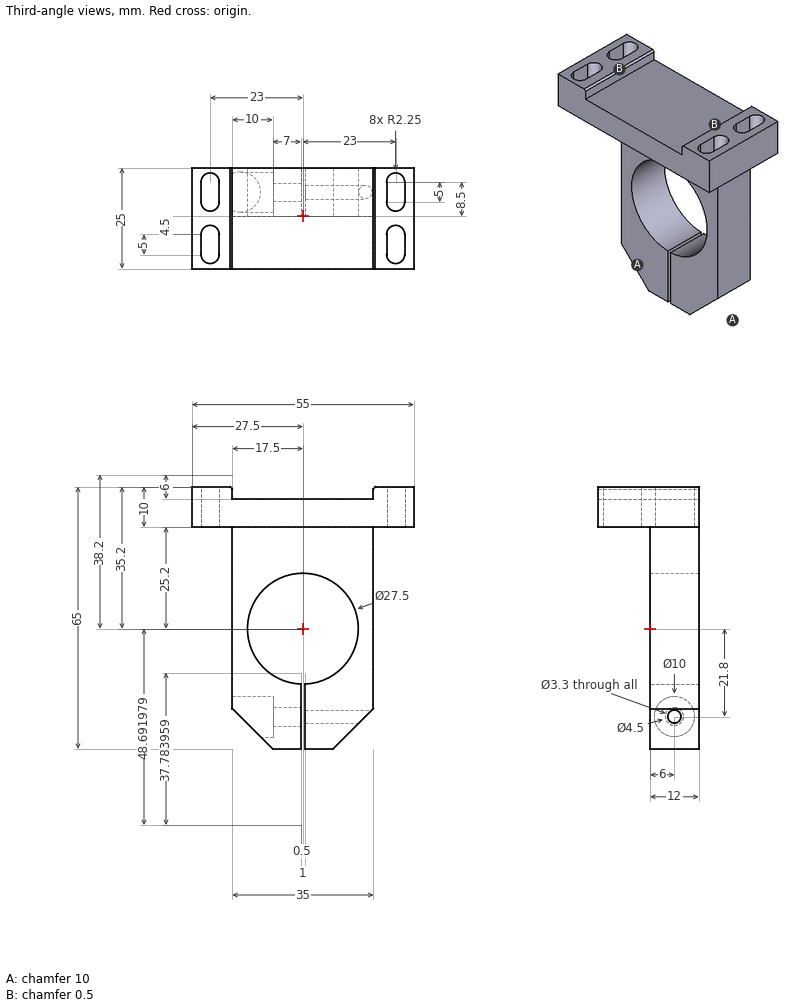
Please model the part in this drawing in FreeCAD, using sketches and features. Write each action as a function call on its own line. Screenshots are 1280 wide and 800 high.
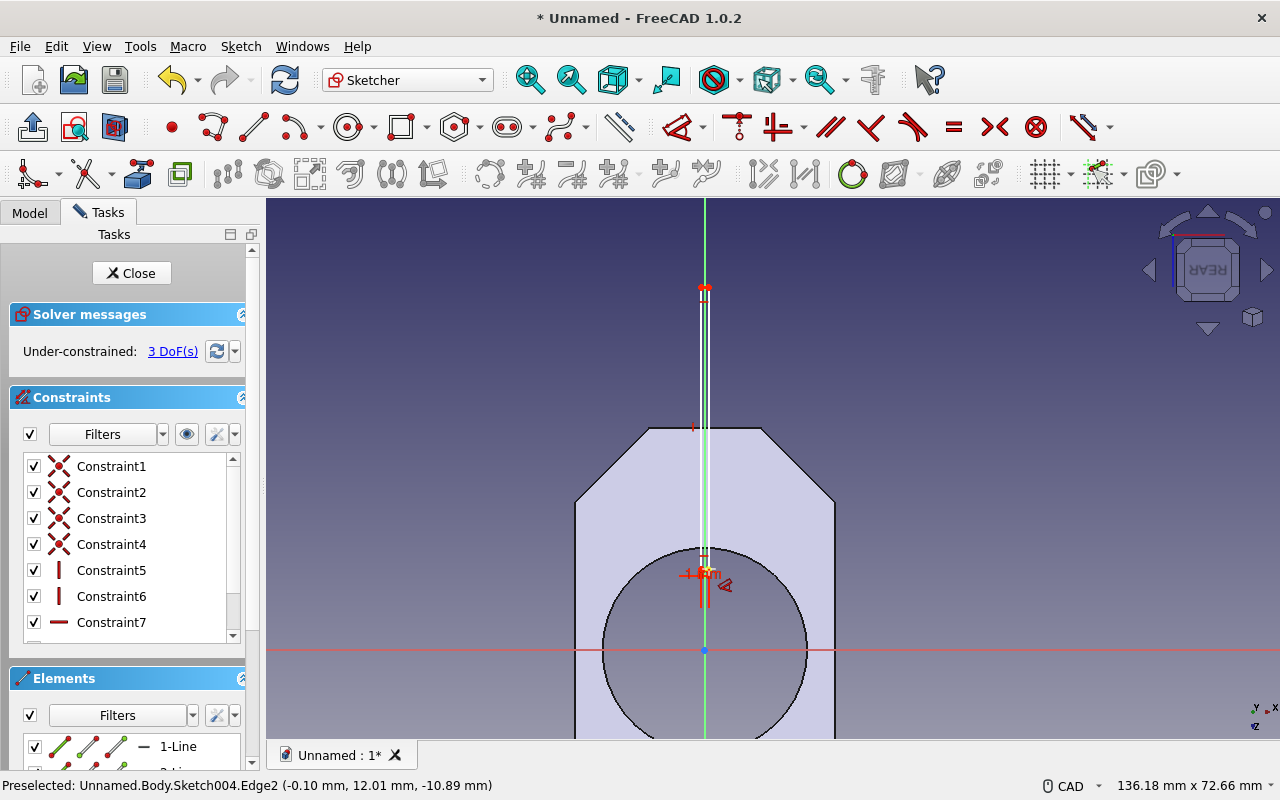
scroll(701, 288, up, 12)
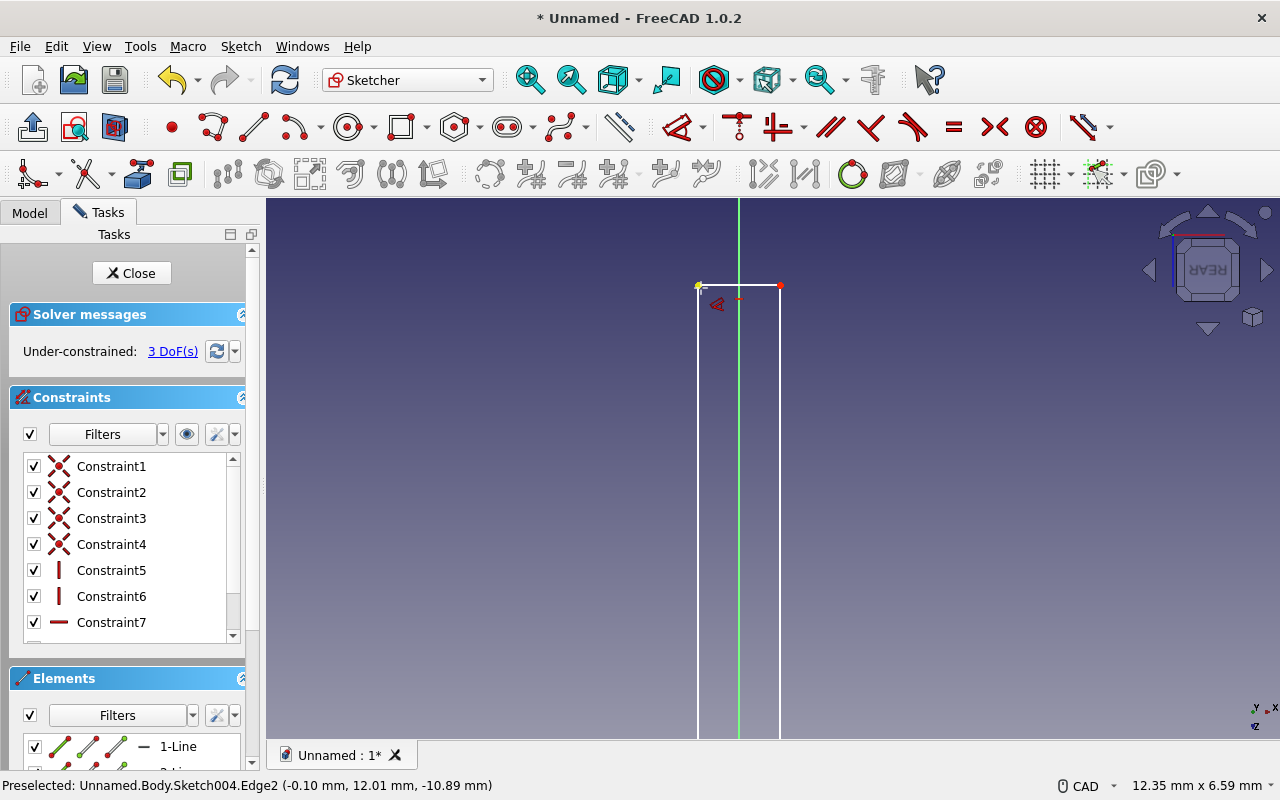
click(698, 285)
click(719, 251)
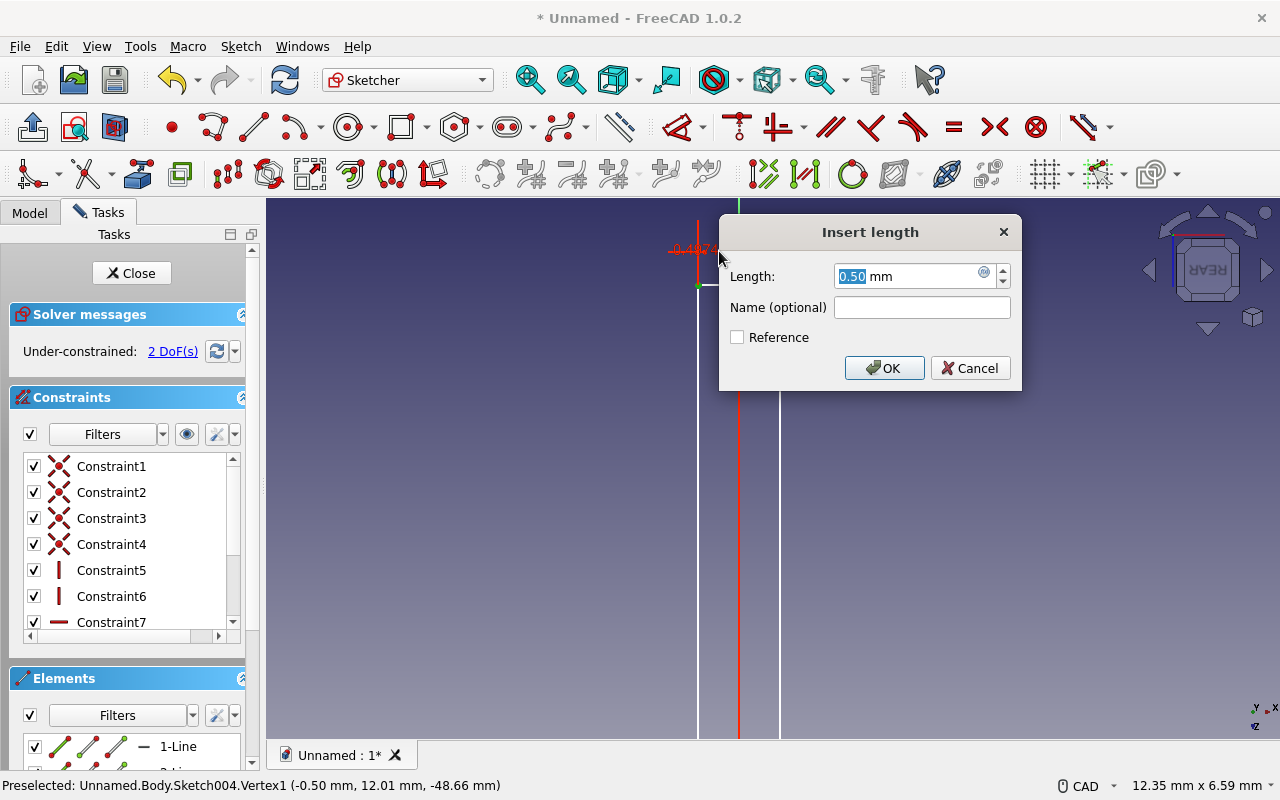
text(0.5)
key(Return)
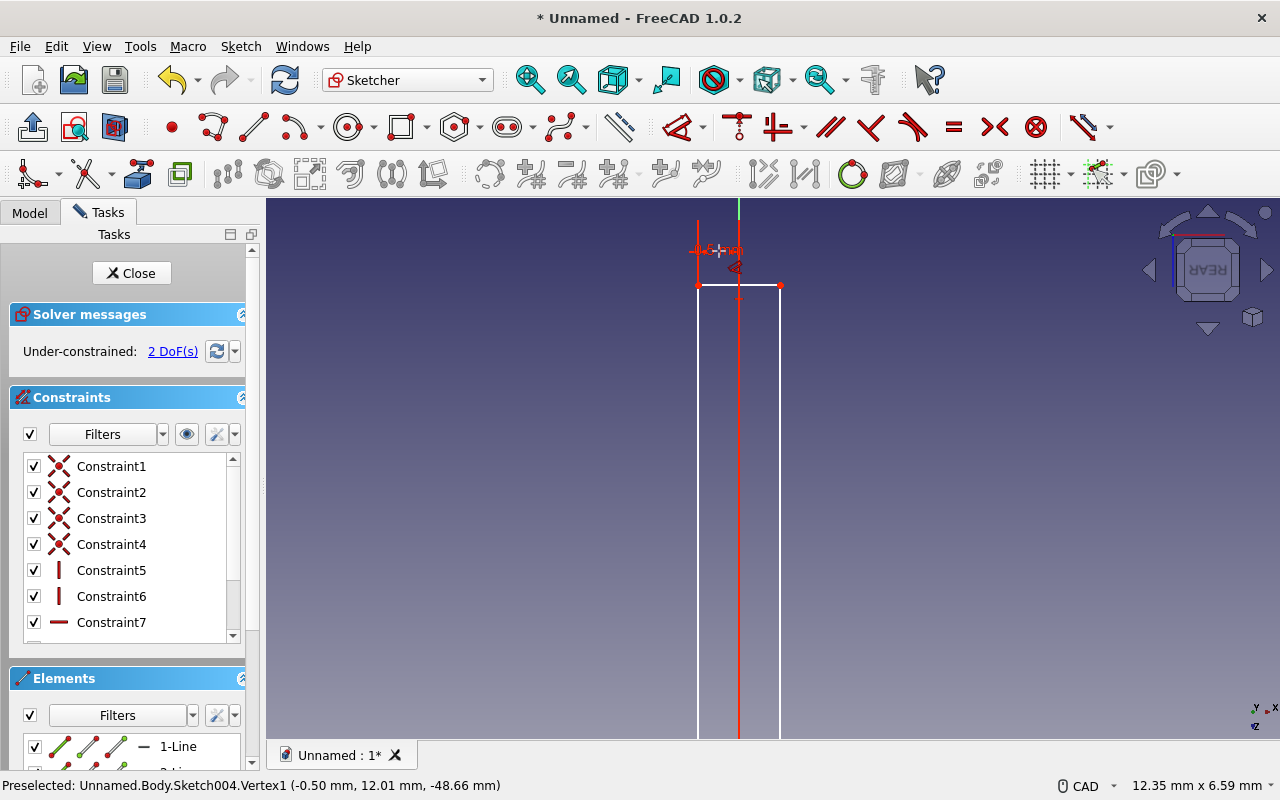
scroll(701, 288, down, 12)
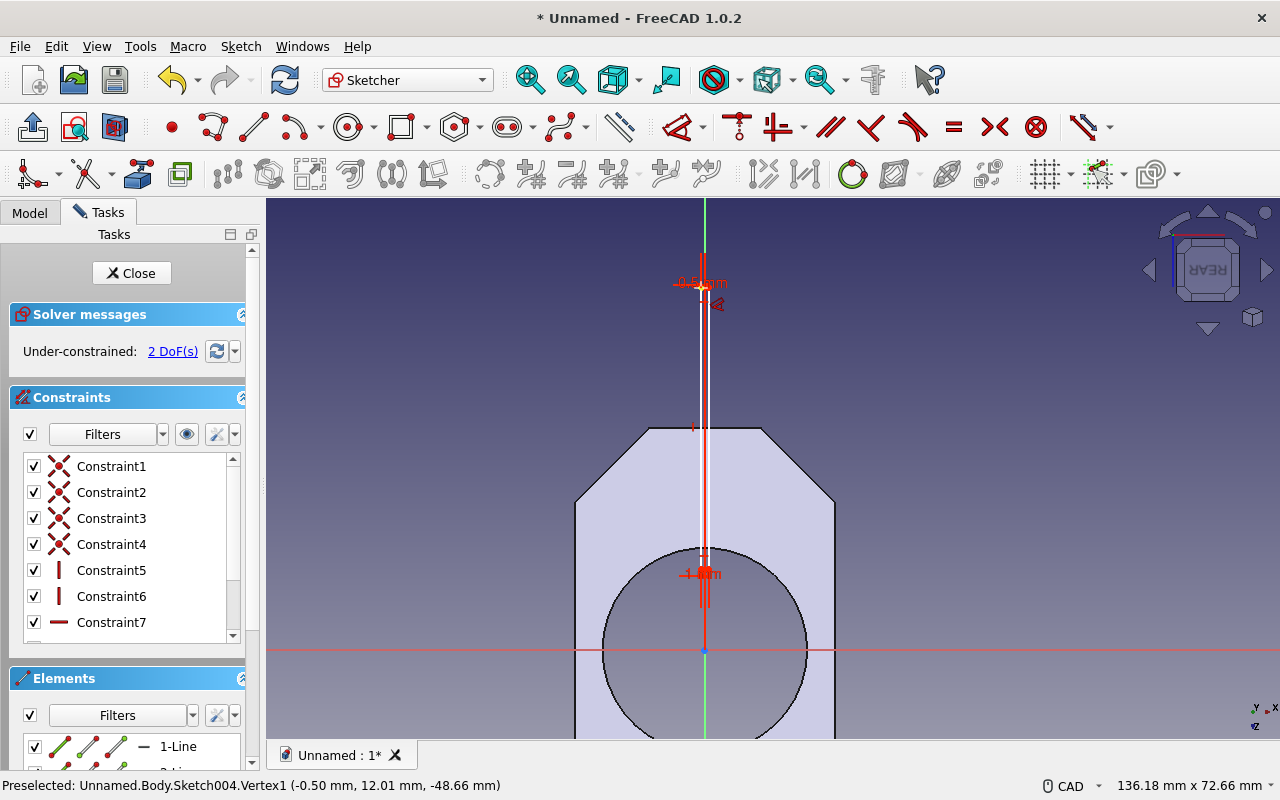
scroll(701, 372, up, 7)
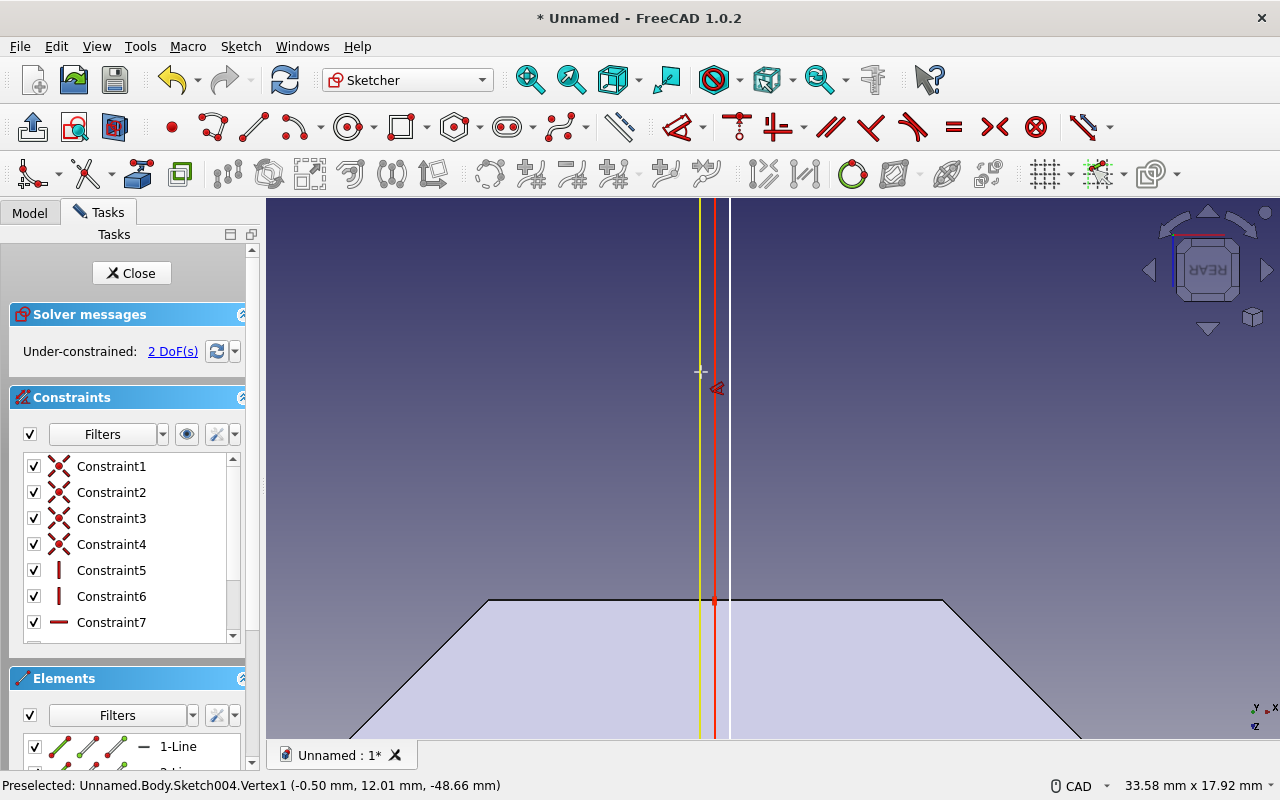
click(700, 372)
click(666, 468)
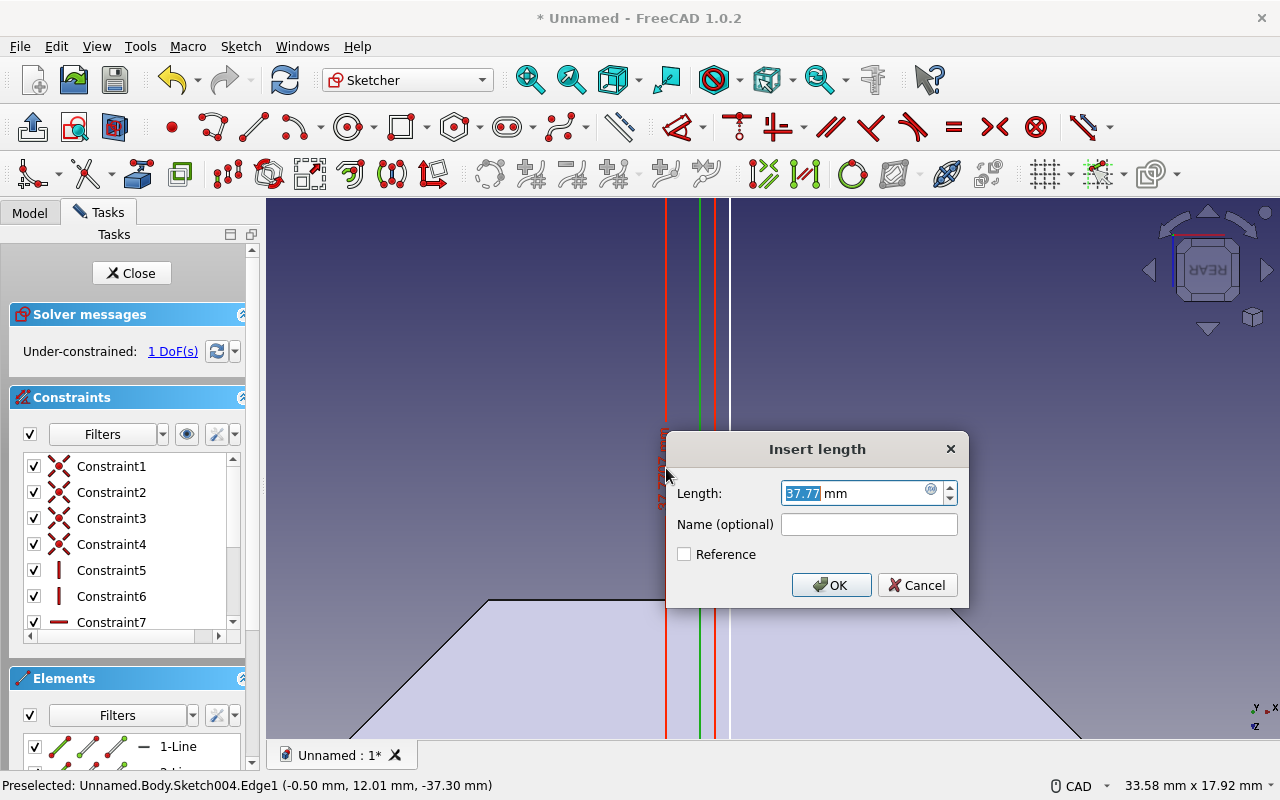
text(37.783959)
key(Return)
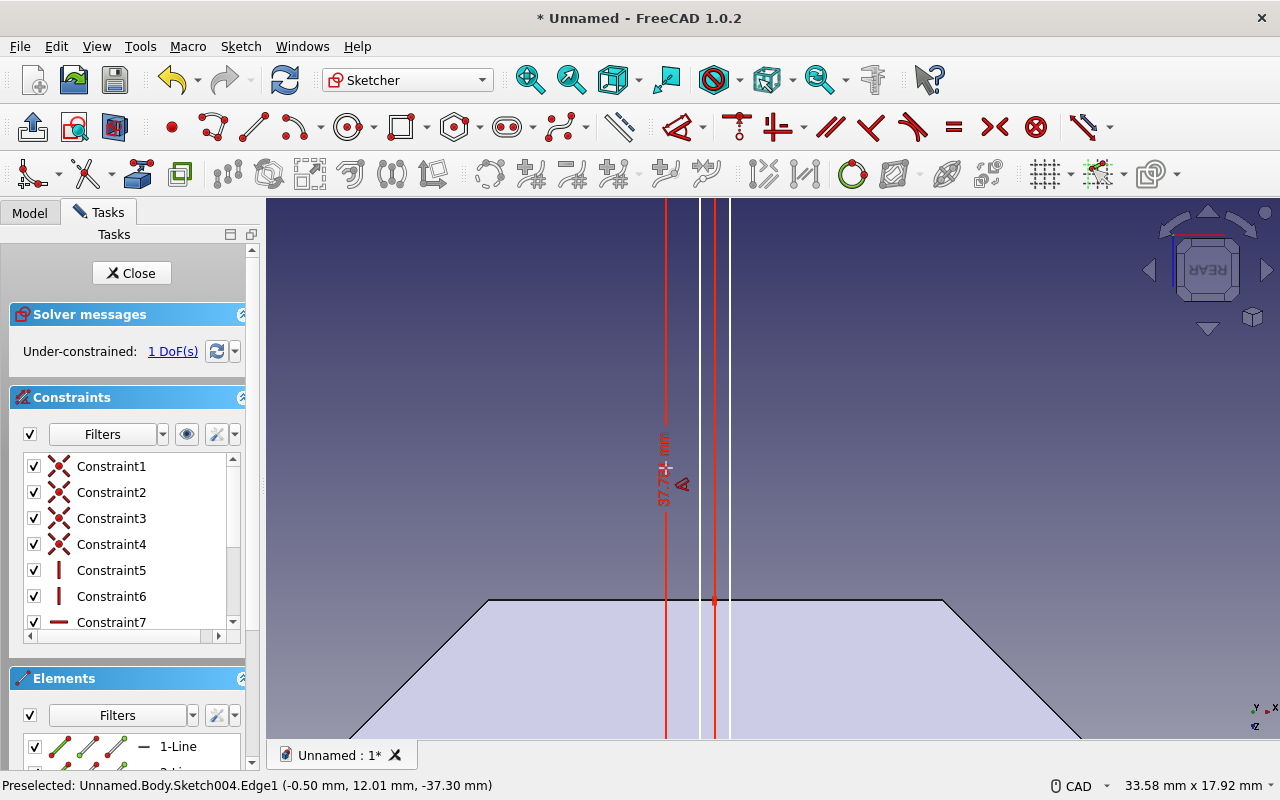
scroll(701, 372, down, 7)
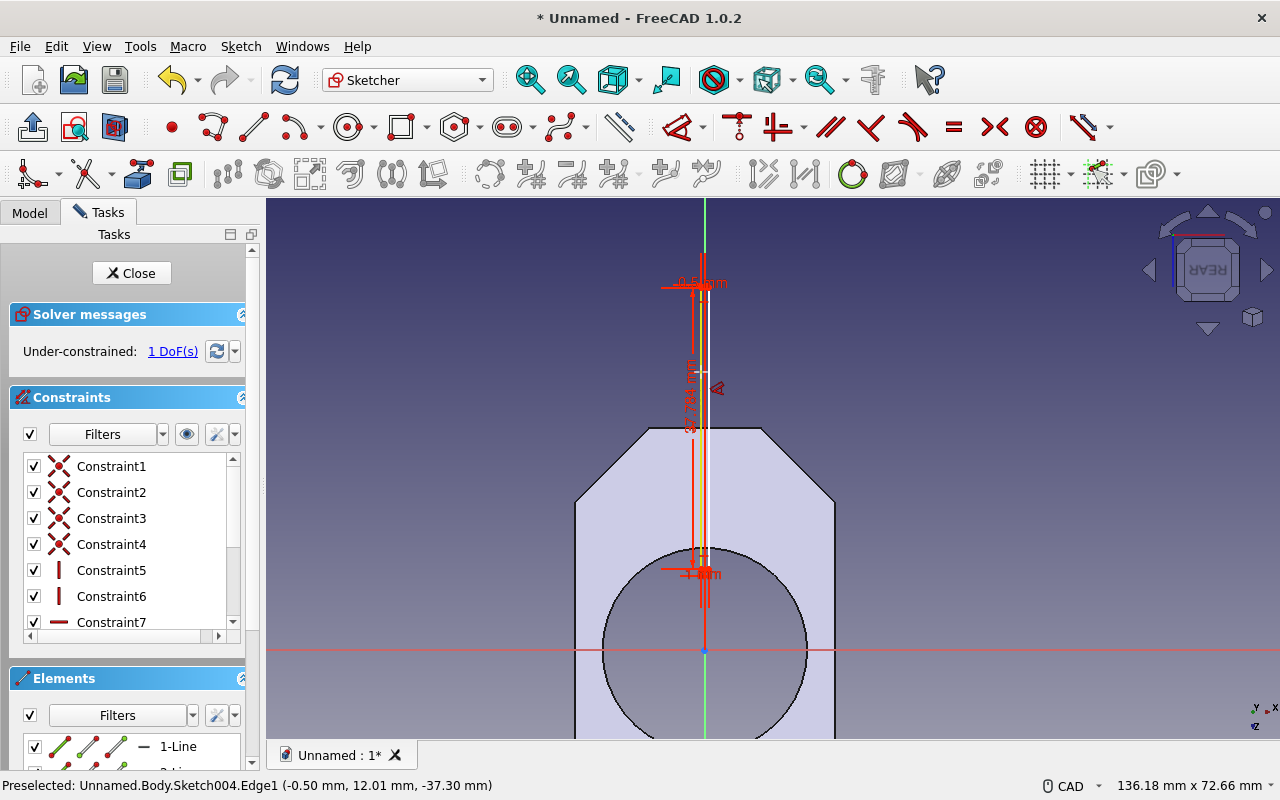
scroll(701, 288, up, 3)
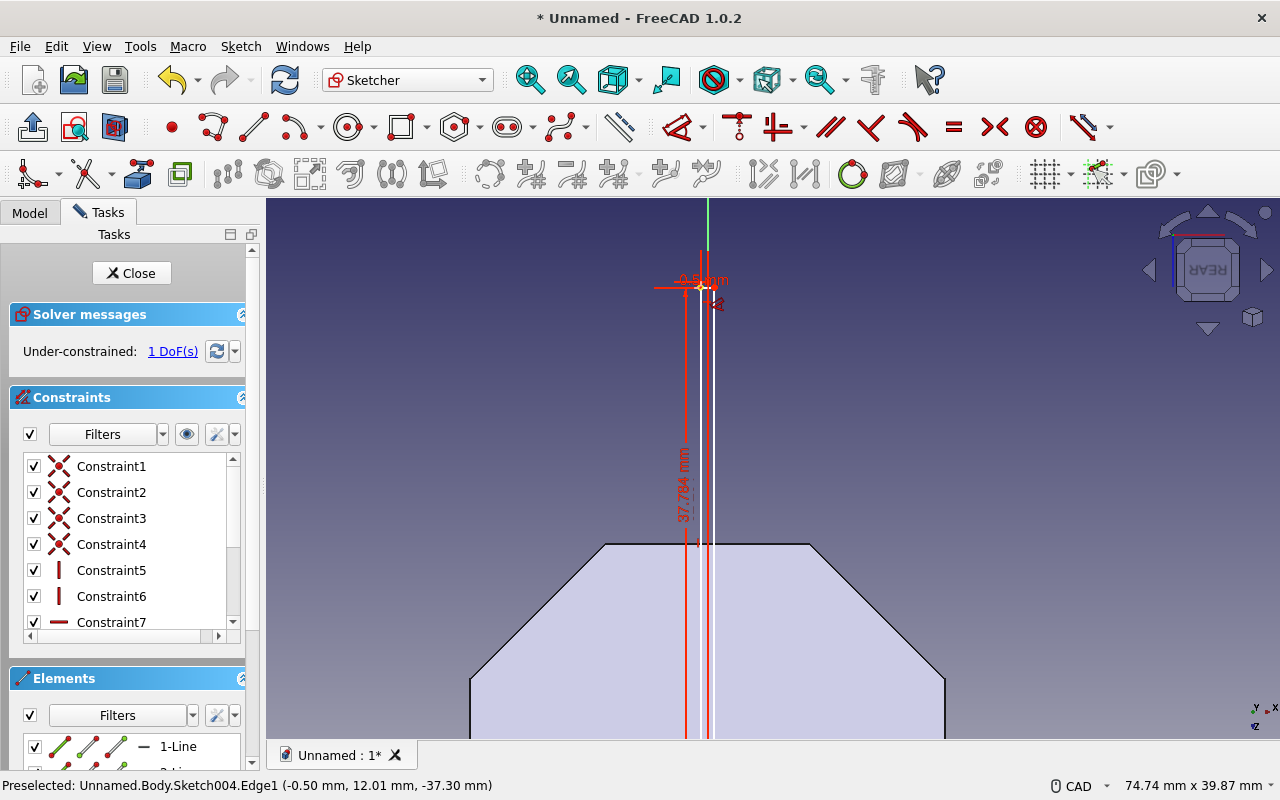
click(701, 288)
click(667, 402)